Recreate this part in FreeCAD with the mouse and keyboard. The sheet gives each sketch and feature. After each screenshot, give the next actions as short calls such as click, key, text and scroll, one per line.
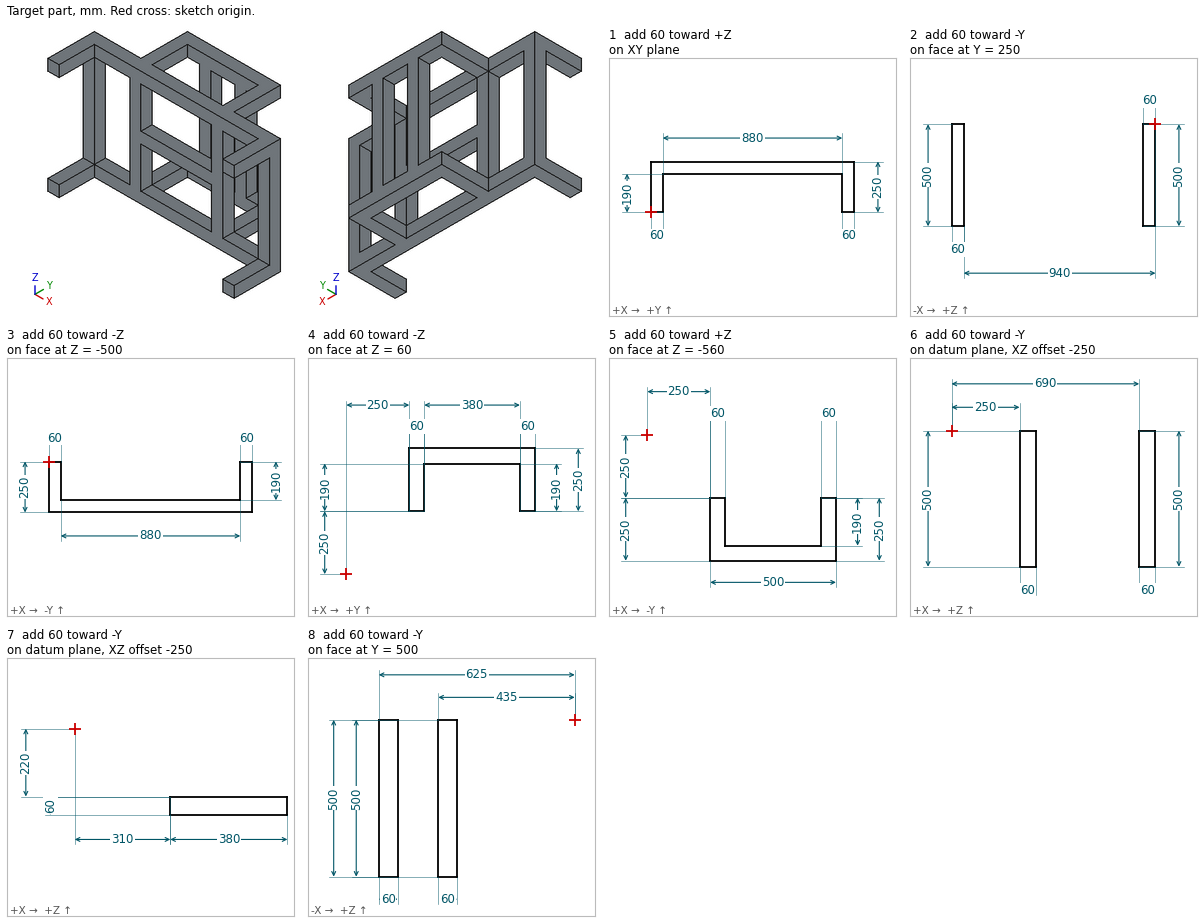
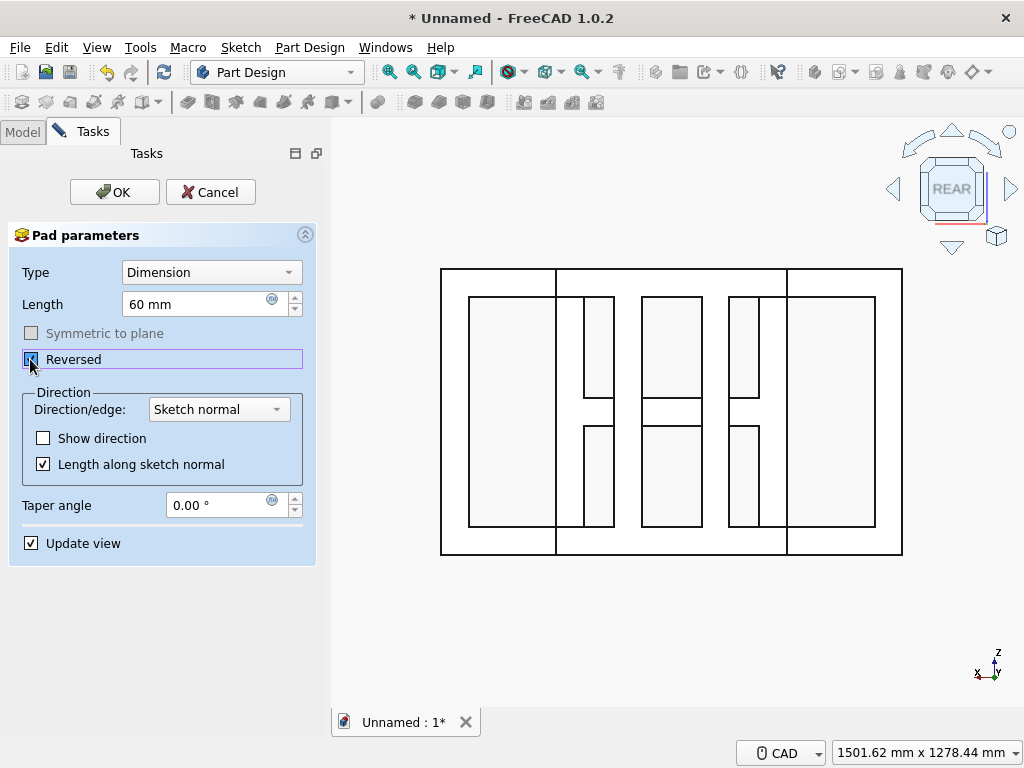
click(115, 192)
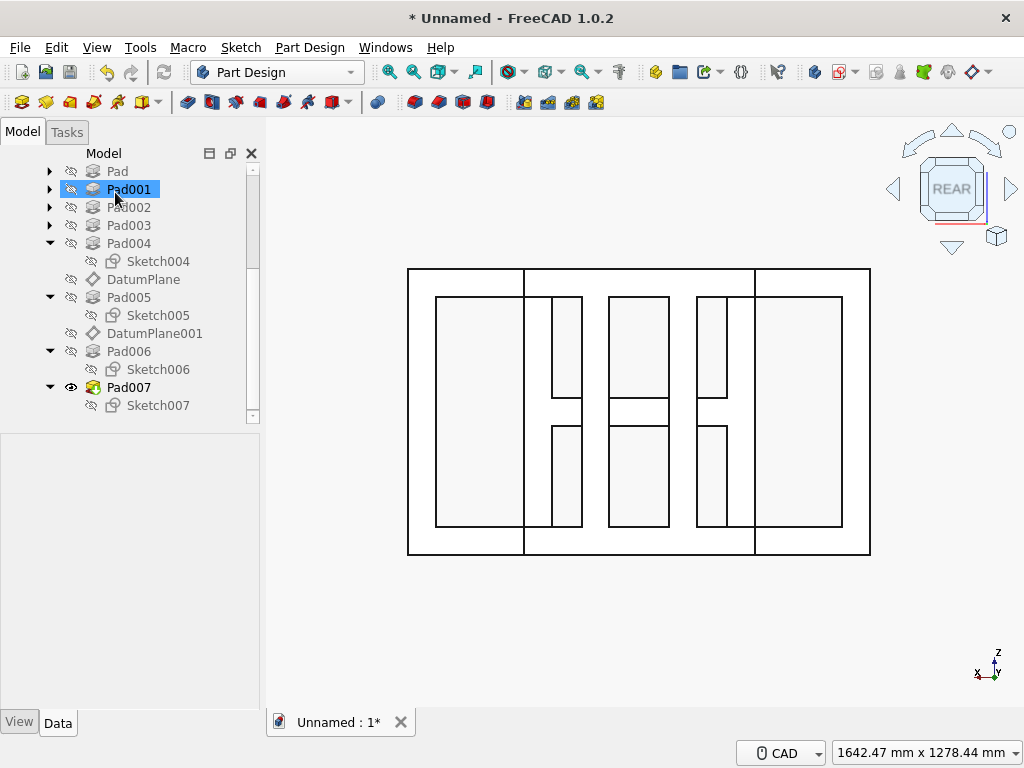
key(0)